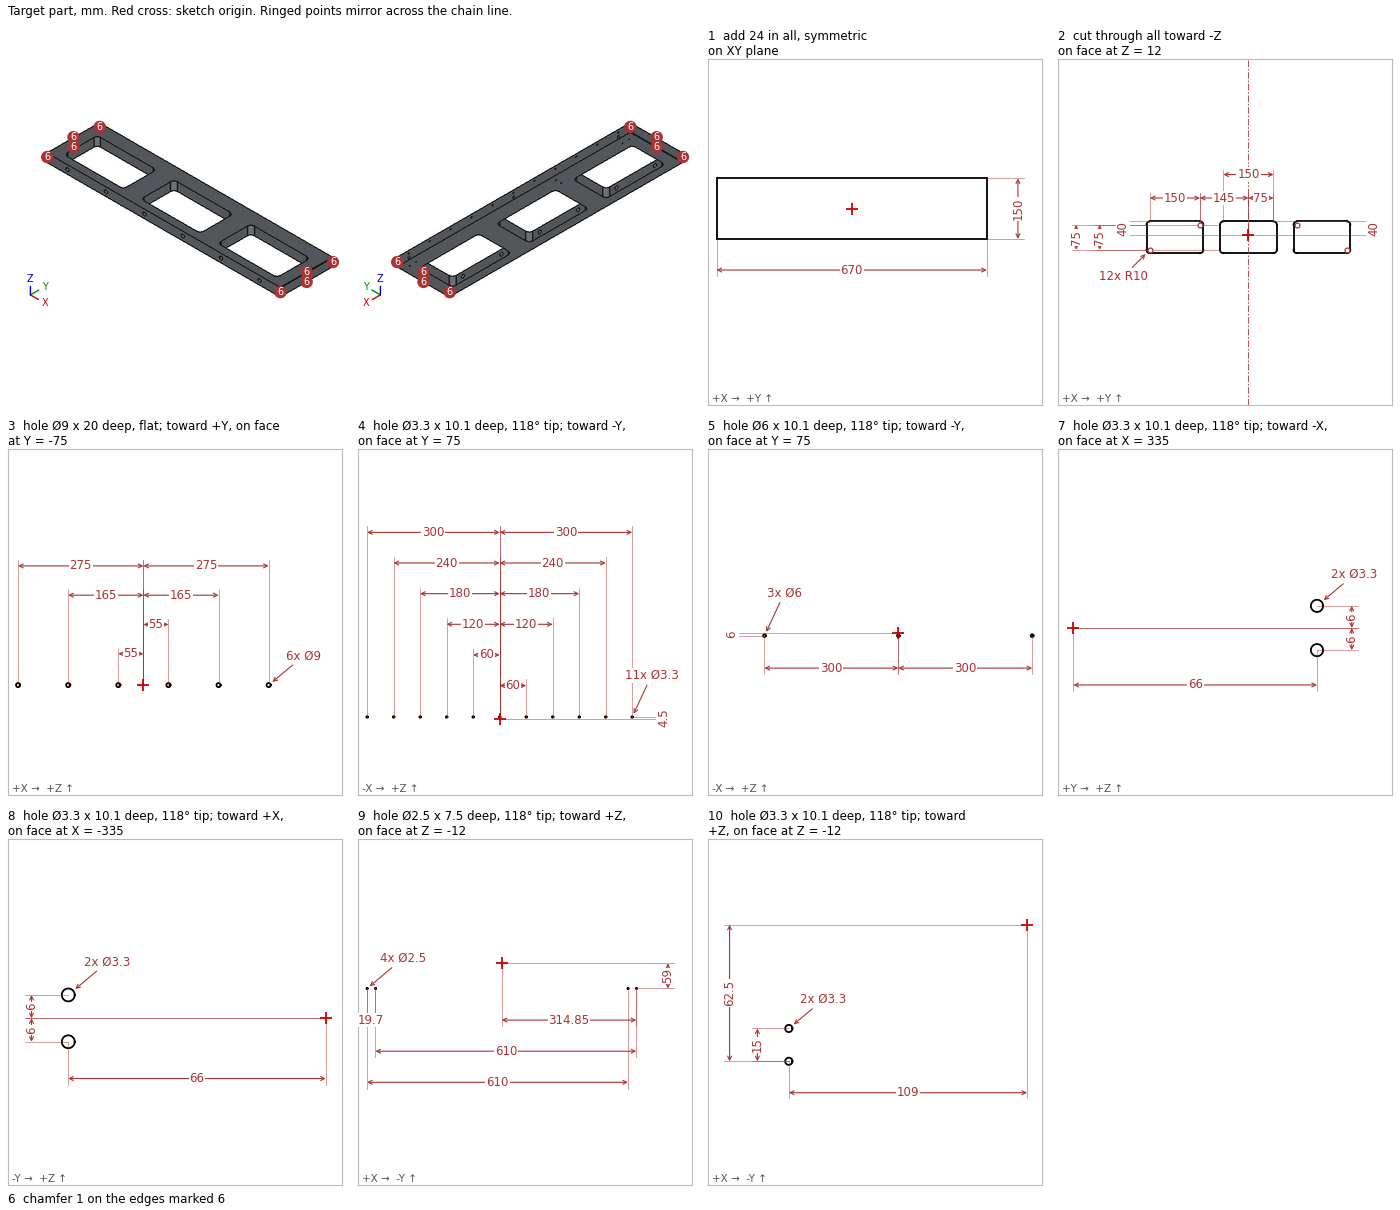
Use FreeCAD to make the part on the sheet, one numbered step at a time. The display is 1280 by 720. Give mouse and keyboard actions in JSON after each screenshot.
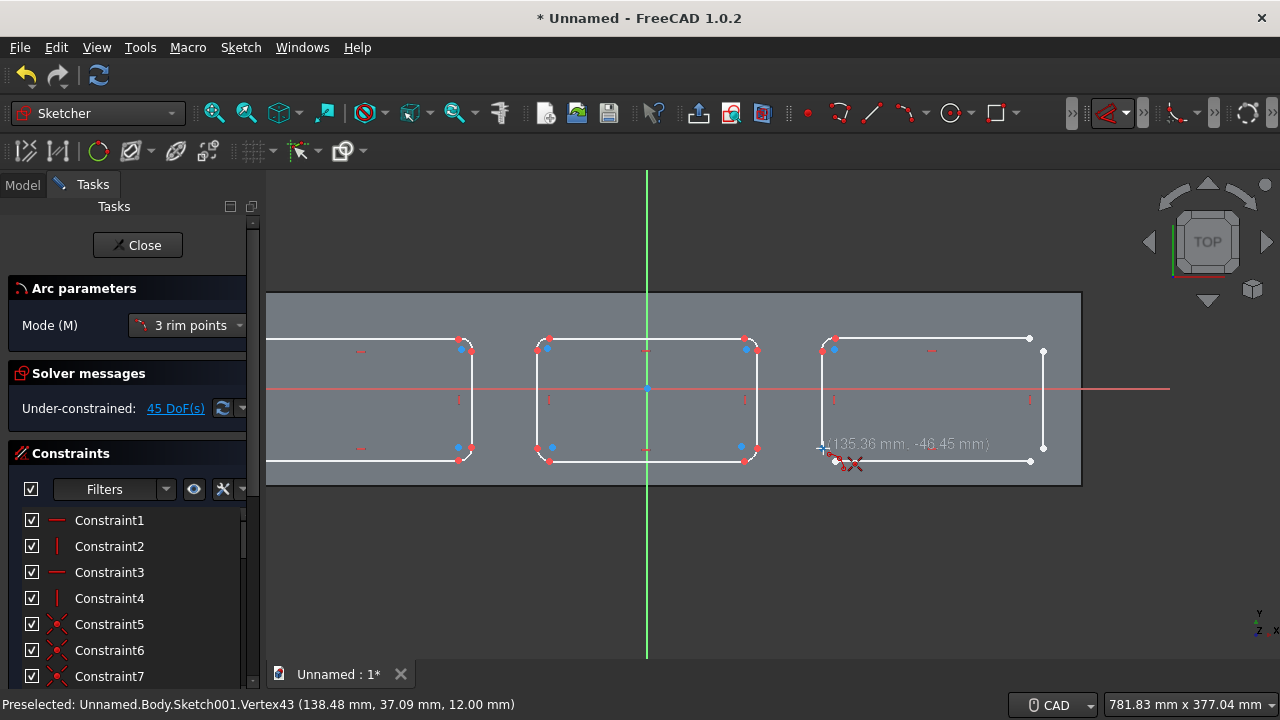
{"action": "left_click", "coordinate": [822, 448]}
{"action": "left_click", "coordinate": [835, 461]}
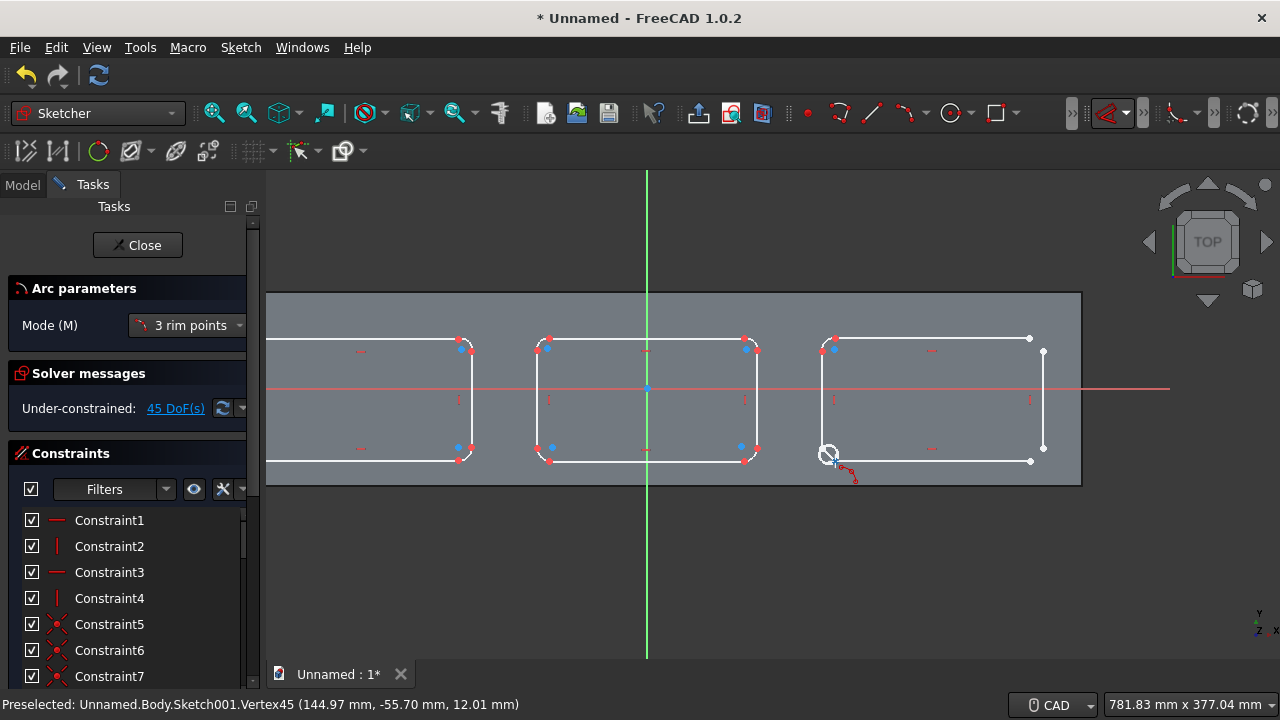
{"action": "scroll", "coordinate": [826, 457], "scroll_direction": "up", "scroll_amount": 8}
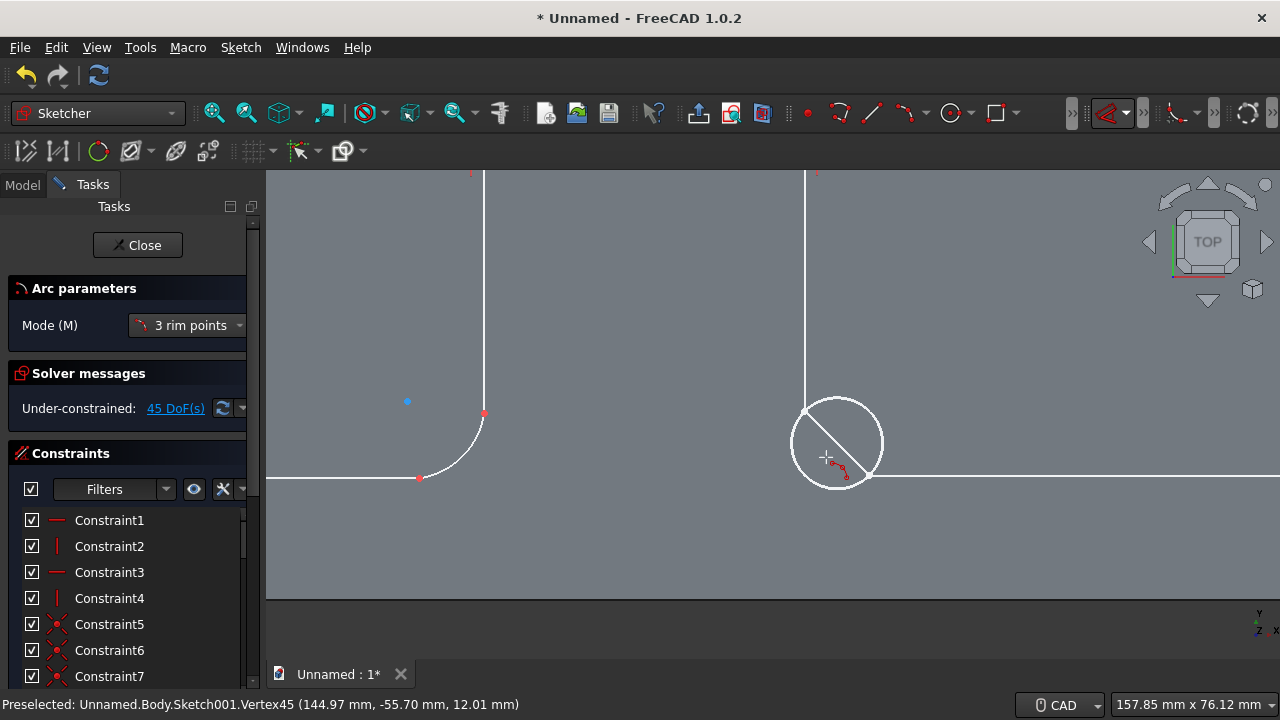
{"action": "left_click", "coordinate": [824, 452]}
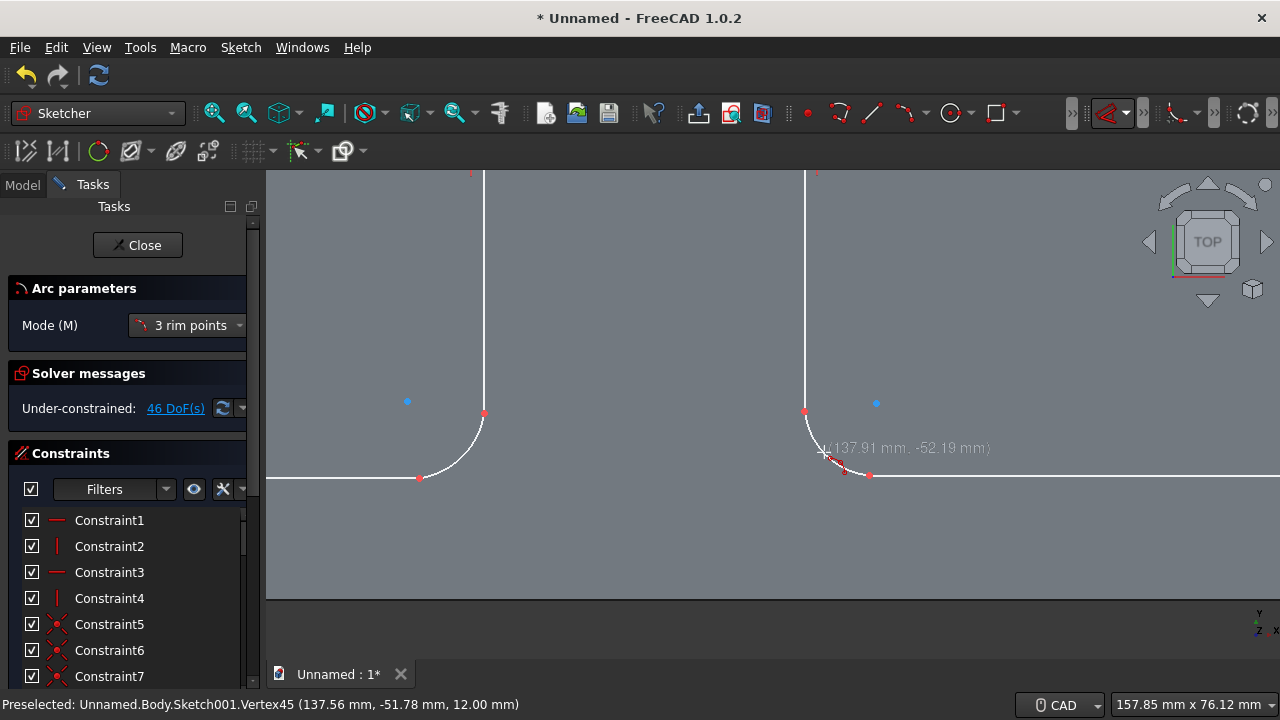
{"action": "scroll", "coordinate": [824, 453], "scroll_direction": "down", "scroll_amount": 10}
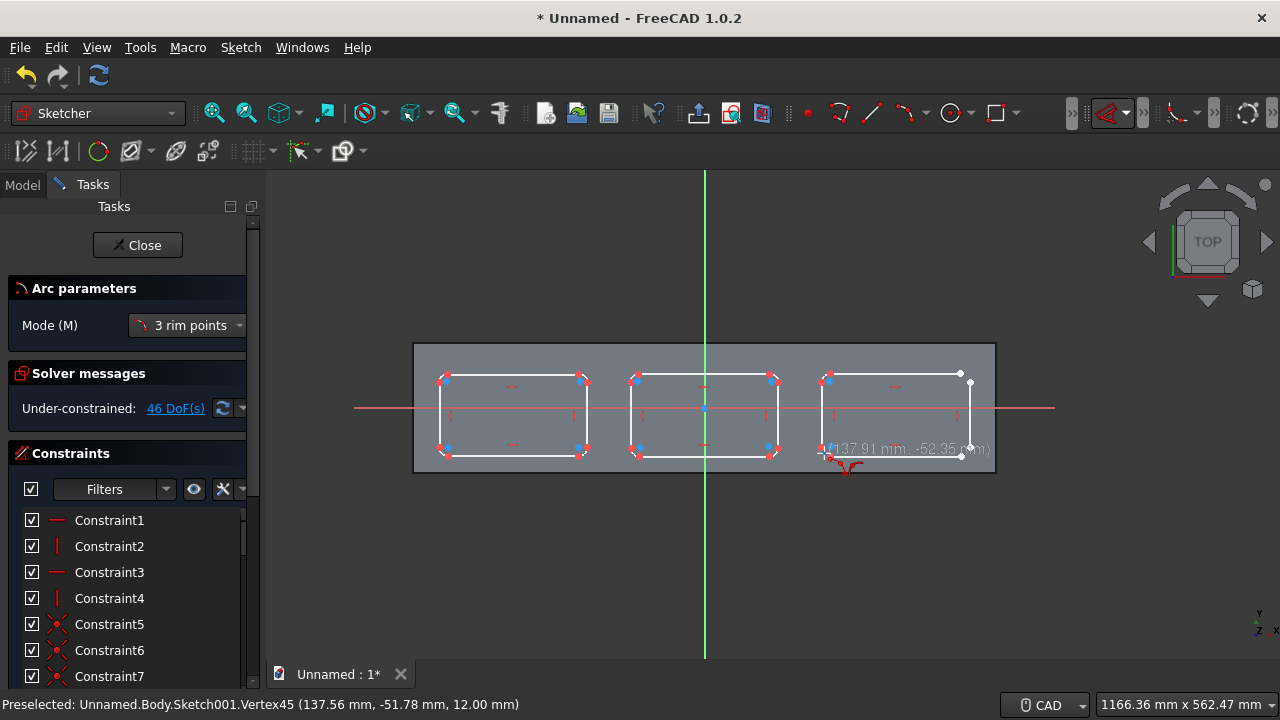
{"action": "scroll", "coordinate": [961, 456], "scroll_direction": "up", "scroll_amount": 2}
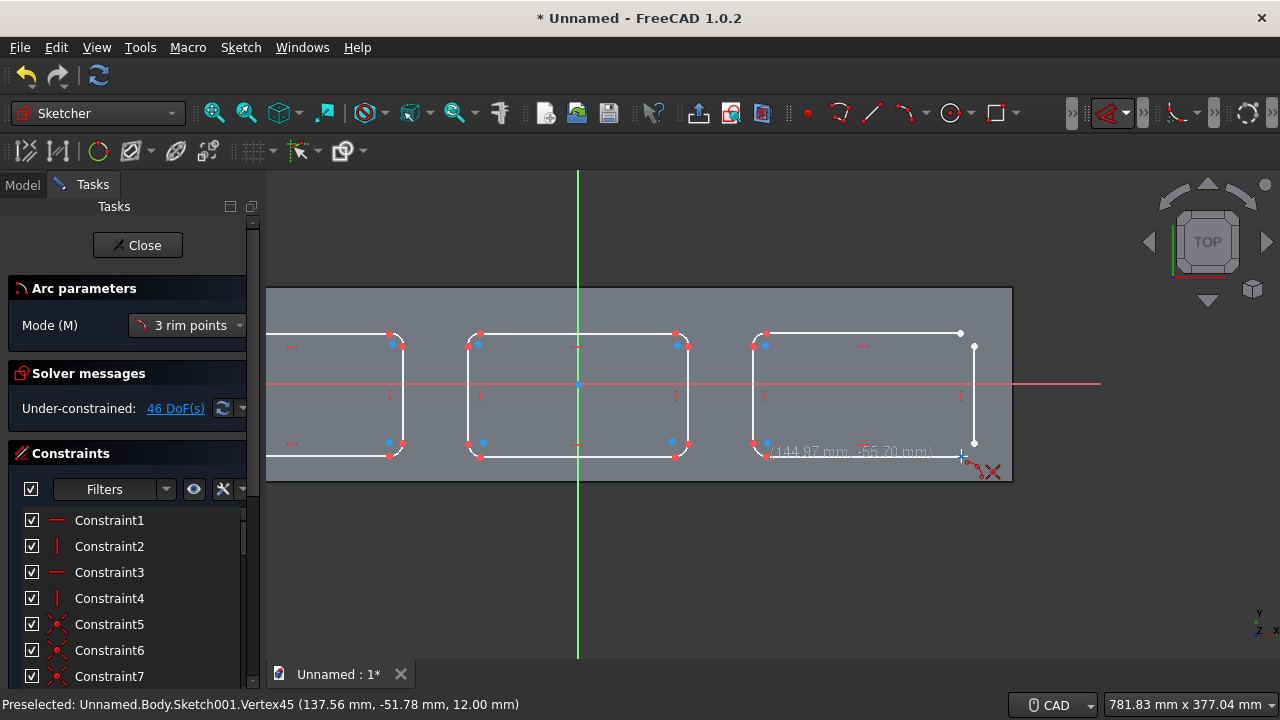
{"action": "left_click", "coordinate": [961, 457]}
{"action": "left_click", "coordinate": [974, 444]}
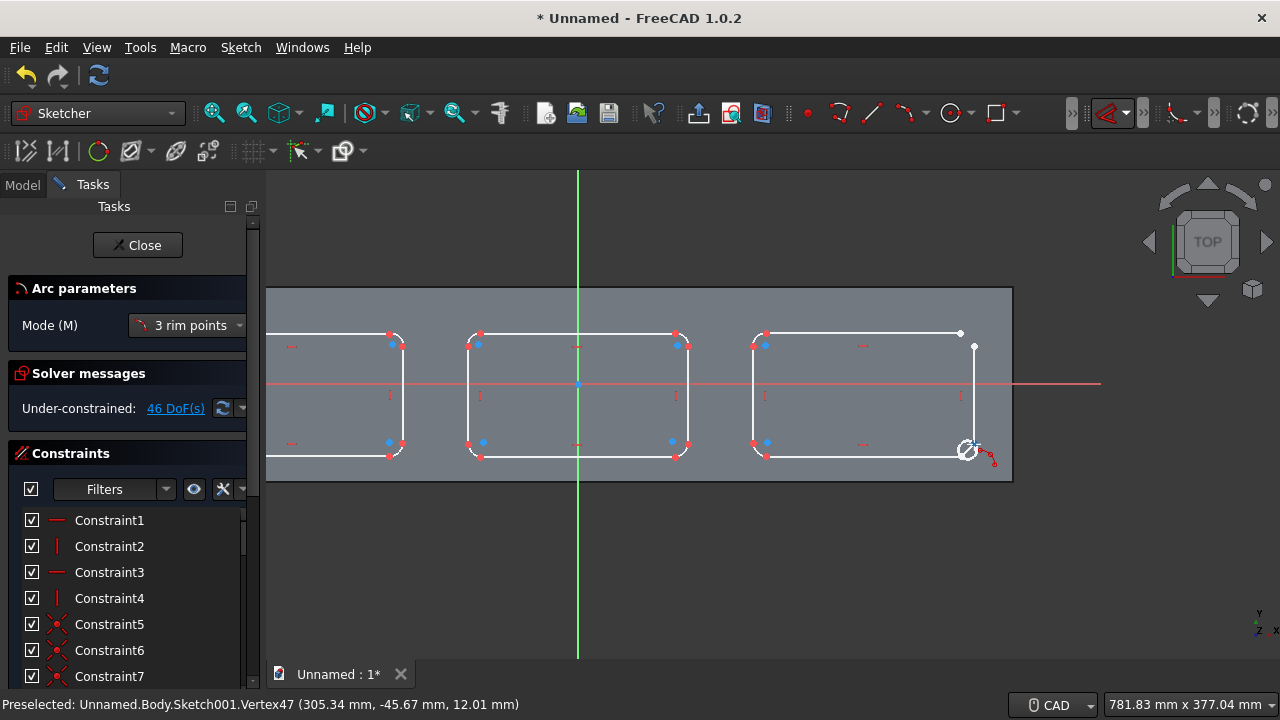
{"action": "scroll", "coordinate": [970, 452], "scroll_direction": "up", "scroll_amount": 8}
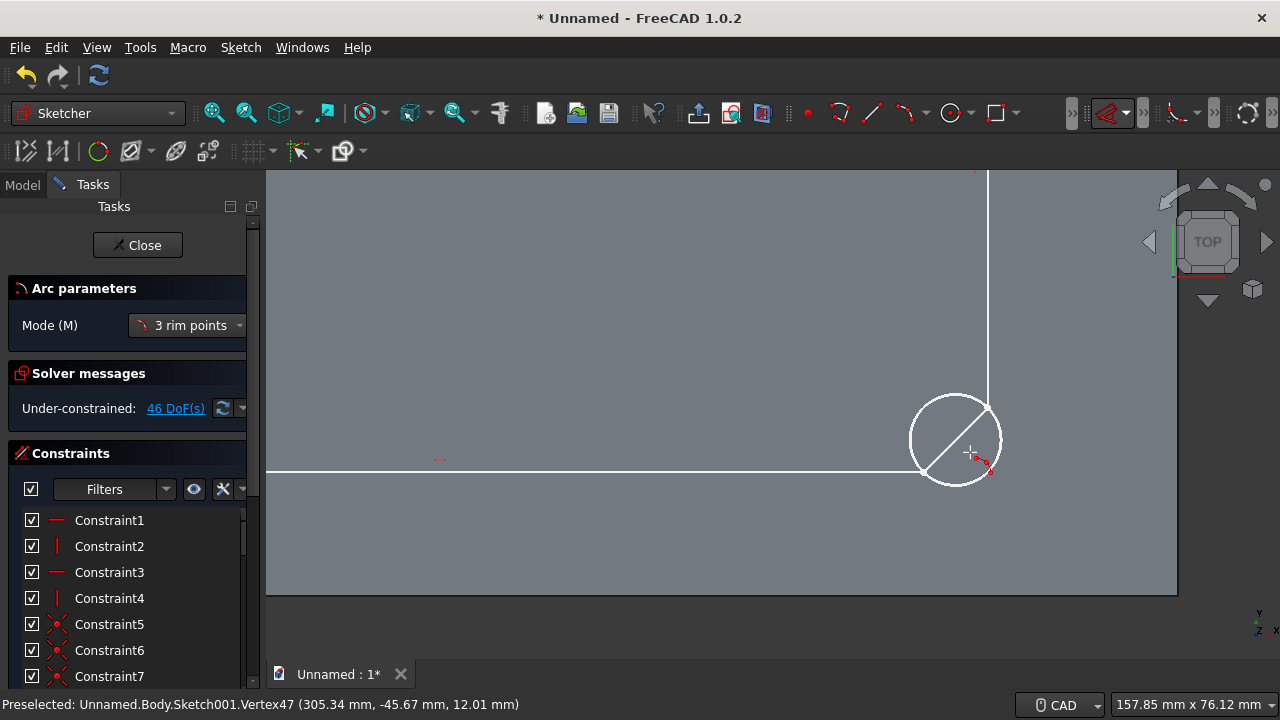
{"action": "left_click", "coordinate": [967, 449]}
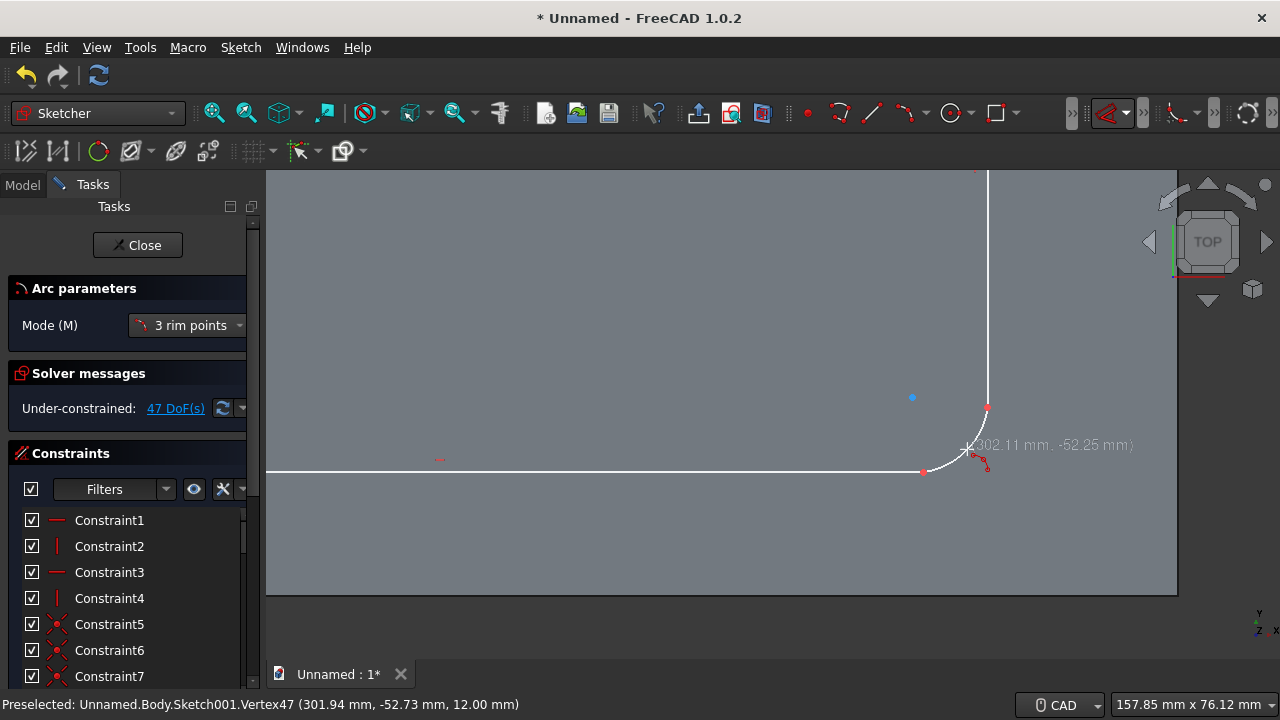
{"action": "scroll", "coordinate": [967, 454], "scroll_direction": "down", "scroll_amount": 10}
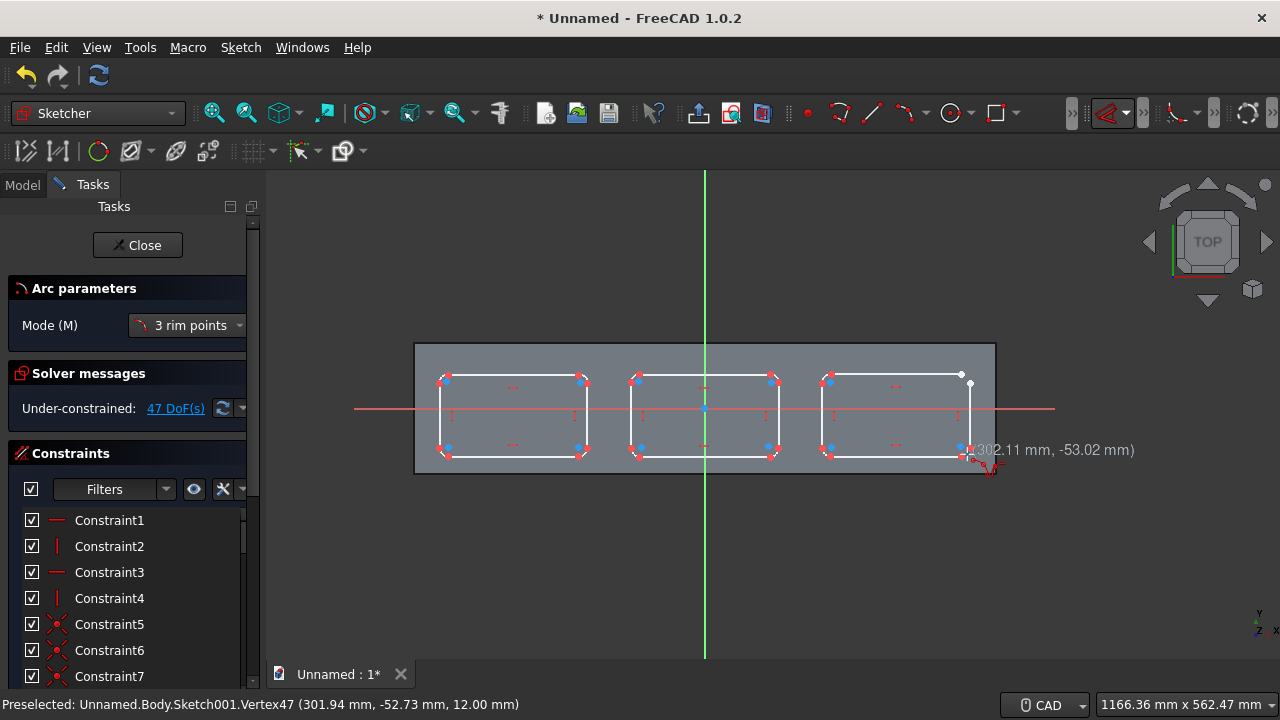
{"action": "scroll", "coordinate": [970, 382], "scroll_direction": "up", "scroll_amount": 2}